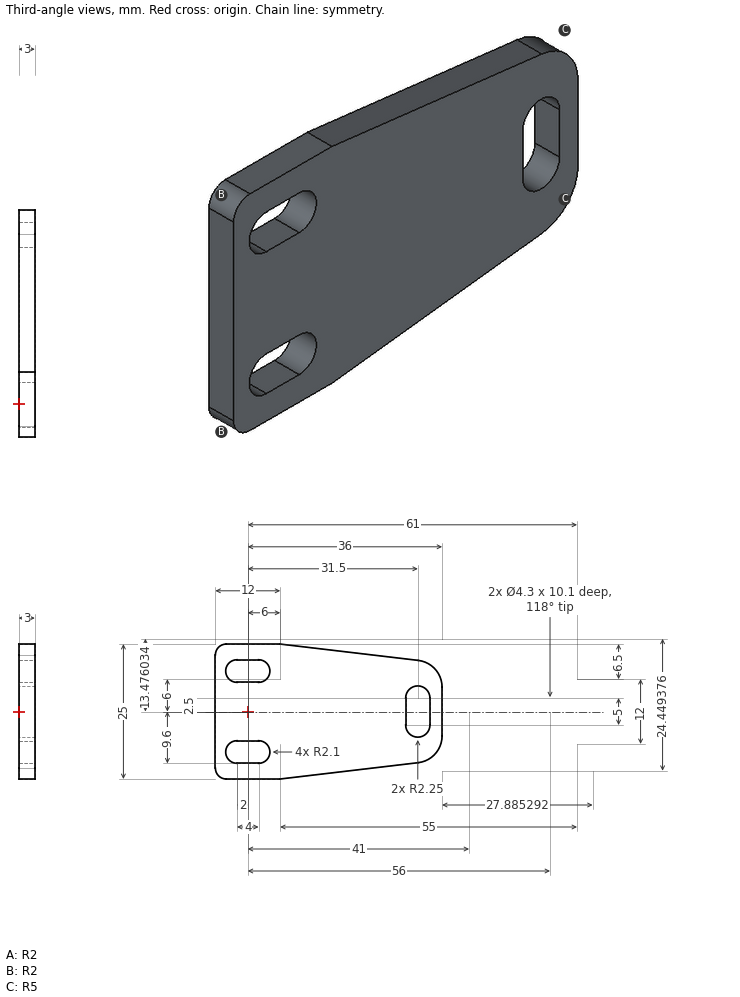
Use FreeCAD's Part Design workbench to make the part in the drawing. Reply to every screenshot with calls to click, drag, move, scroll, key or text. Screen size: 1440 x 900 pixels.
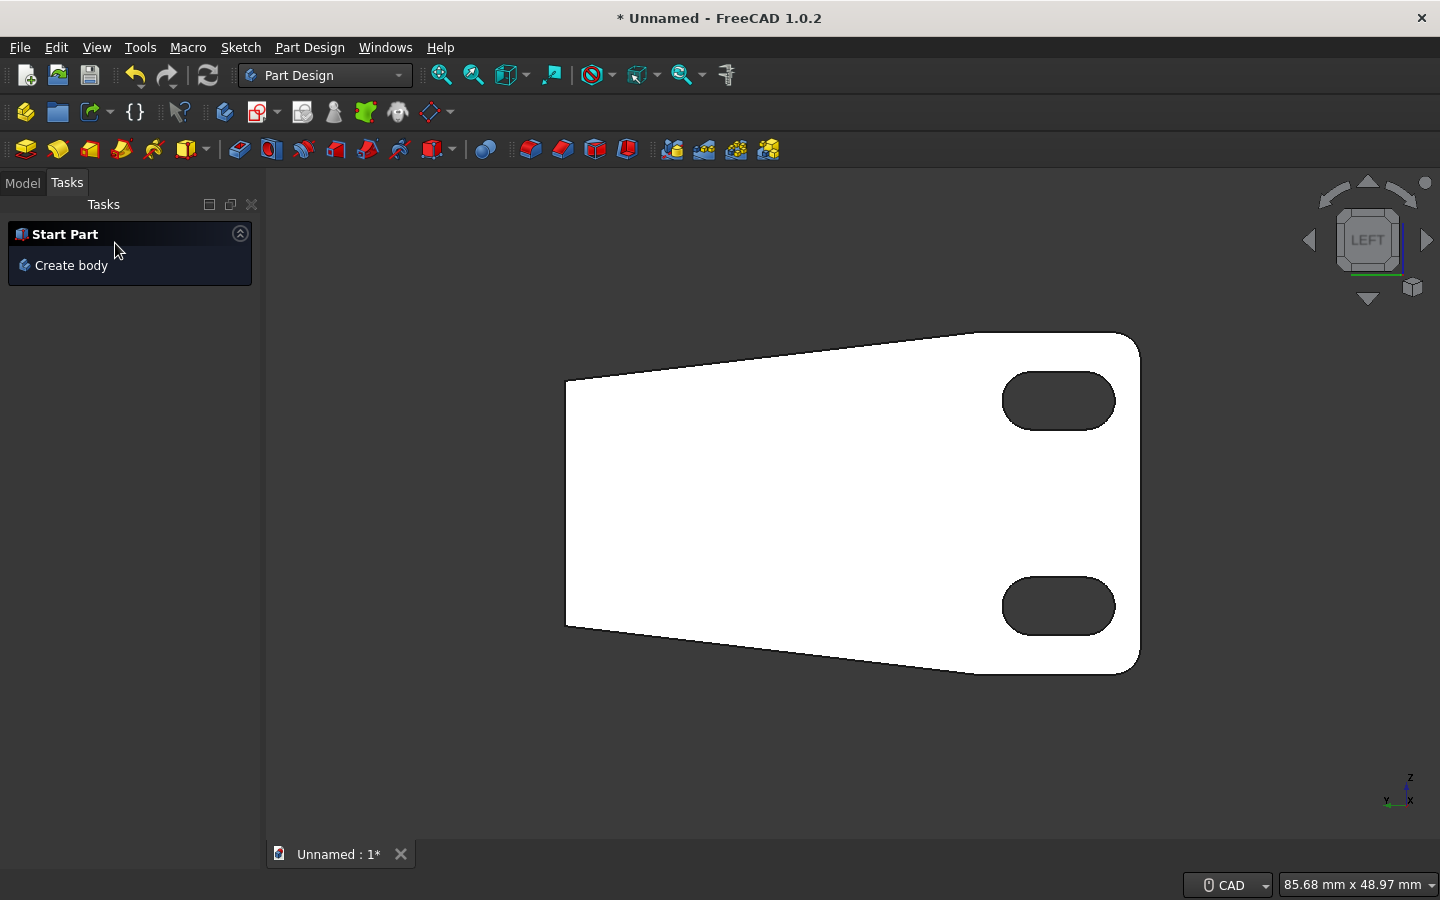
click(853, 502)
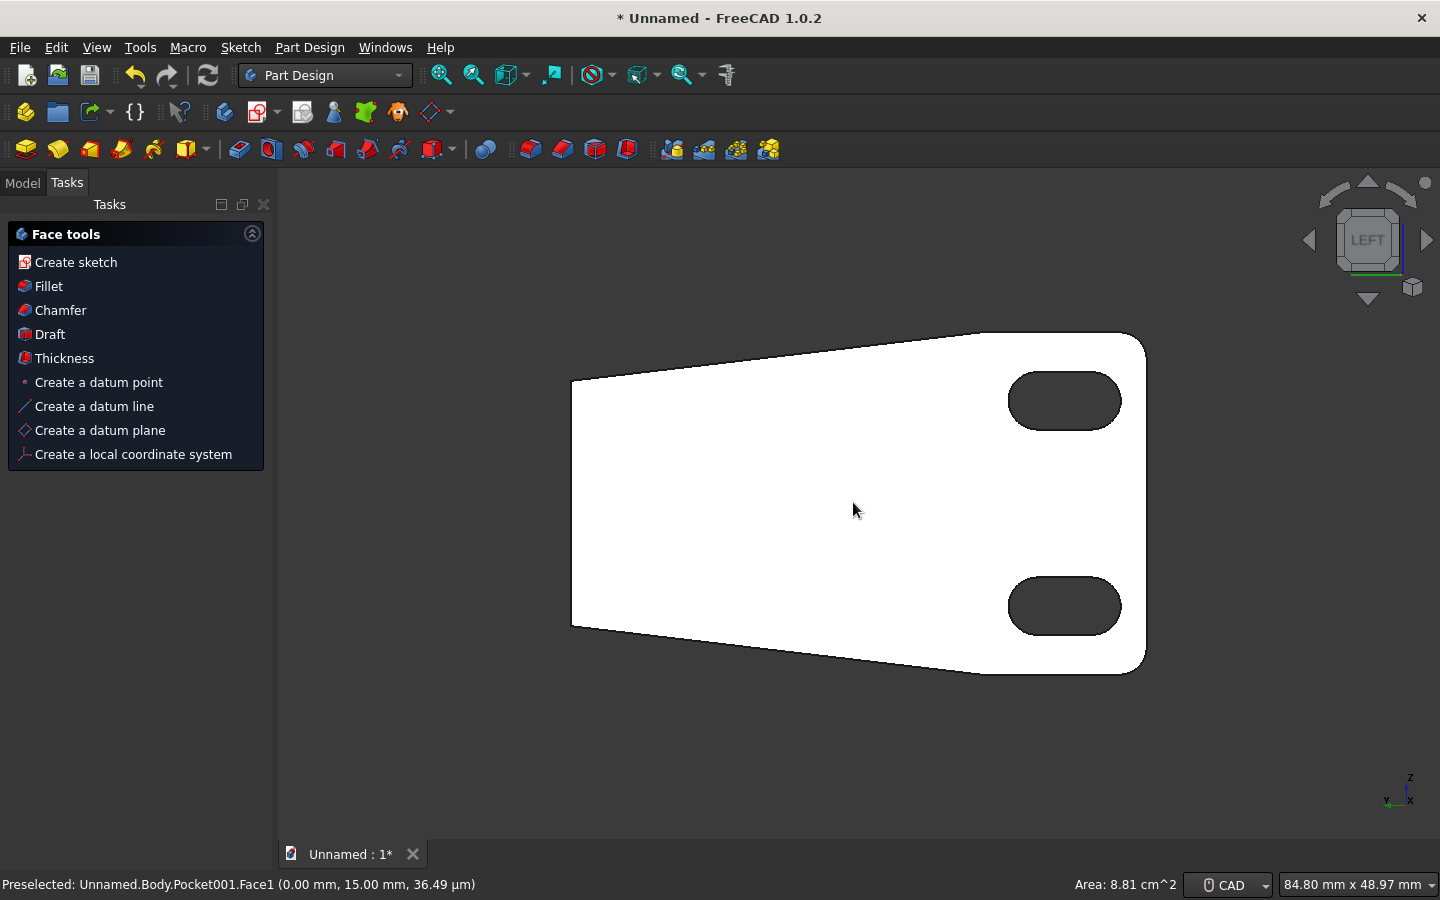
click(258, 112)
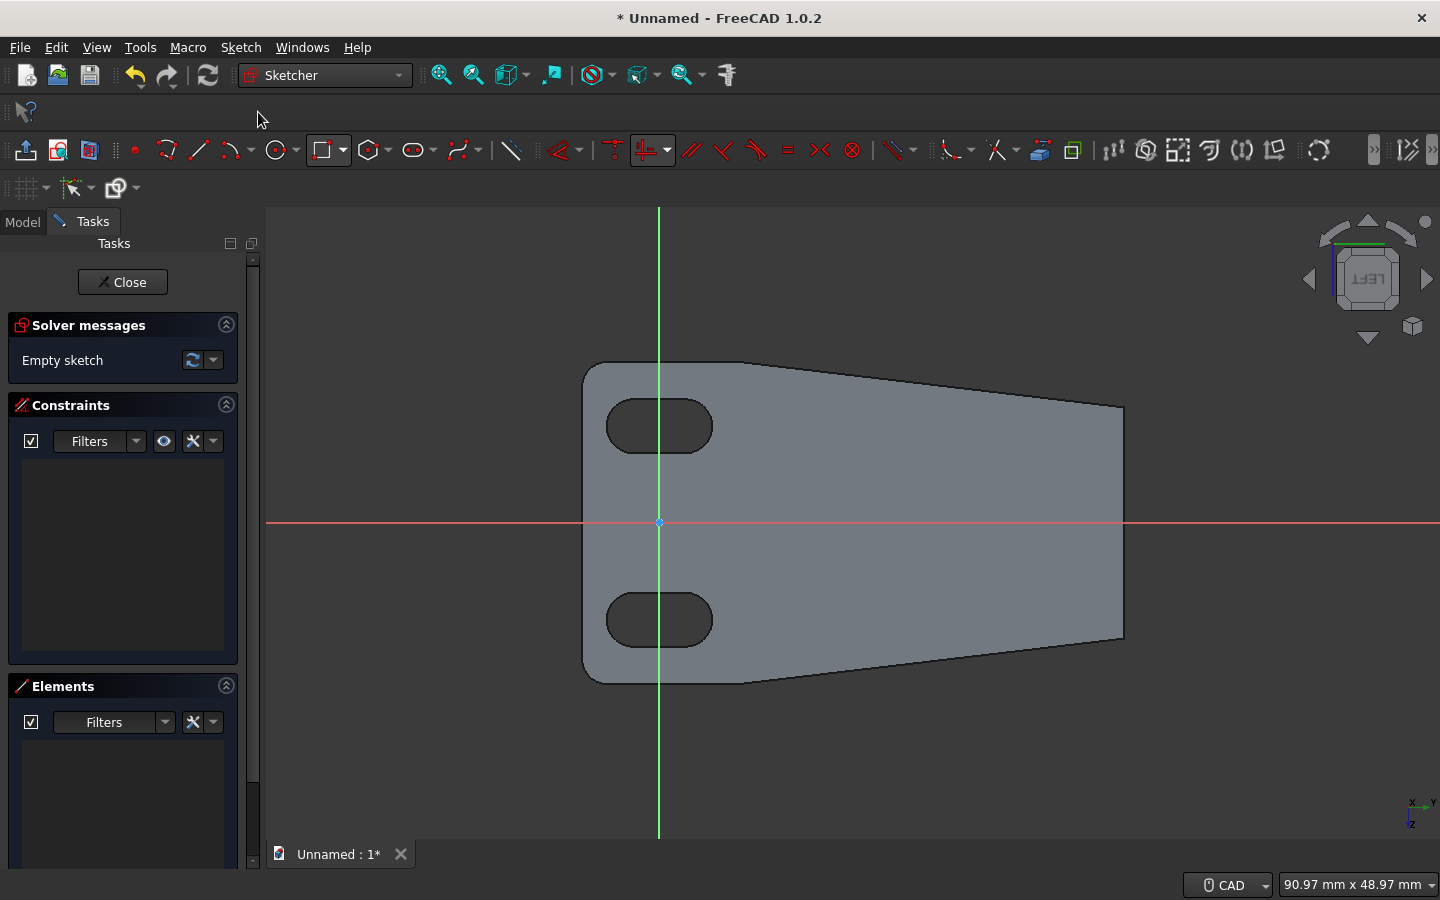
scroll(1187, 523, up, 6)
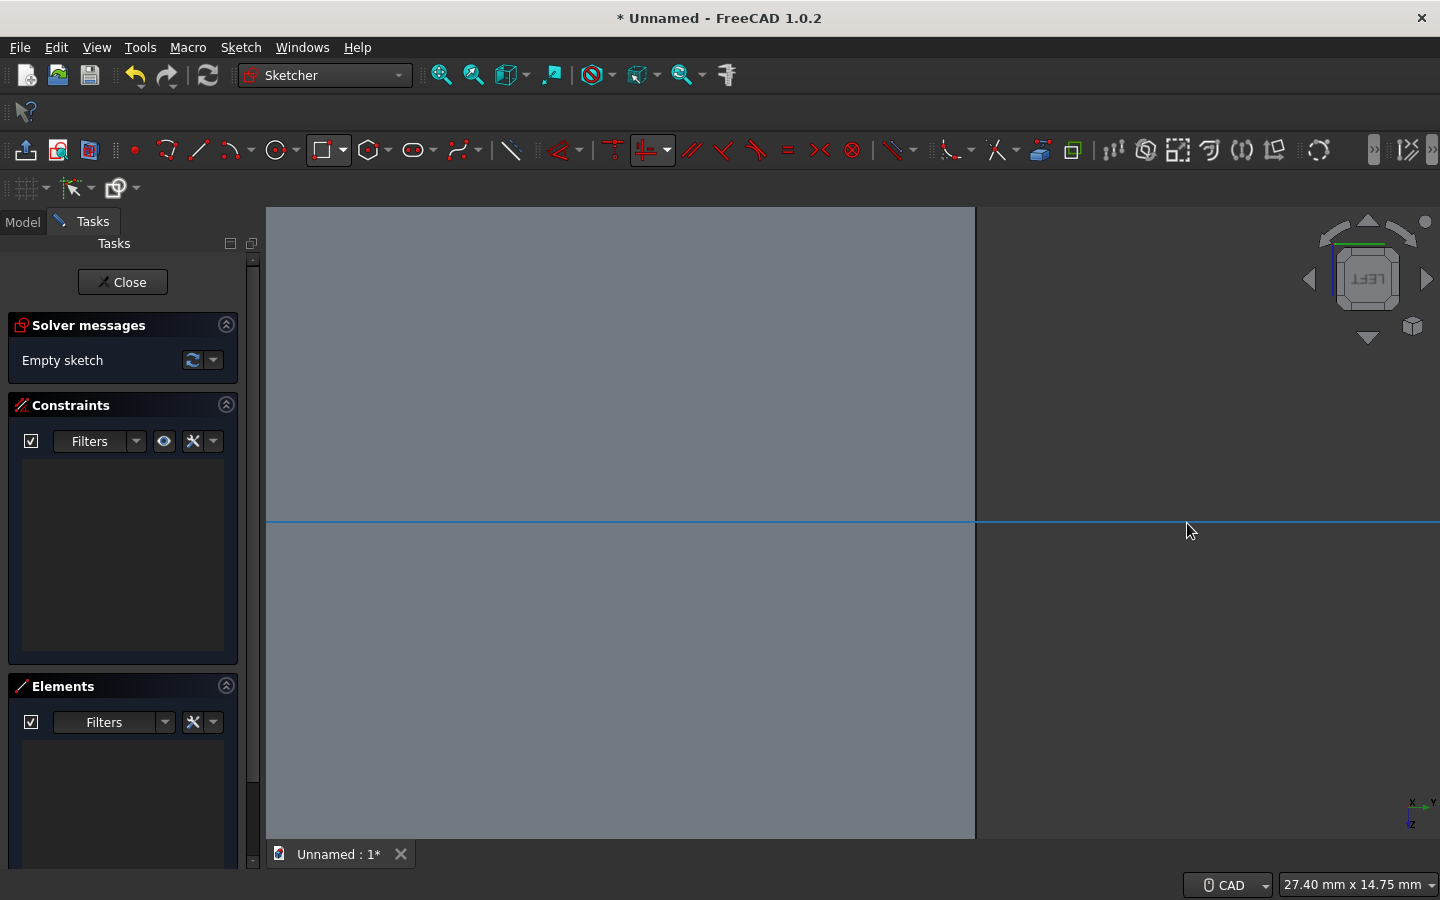
click(414, 150)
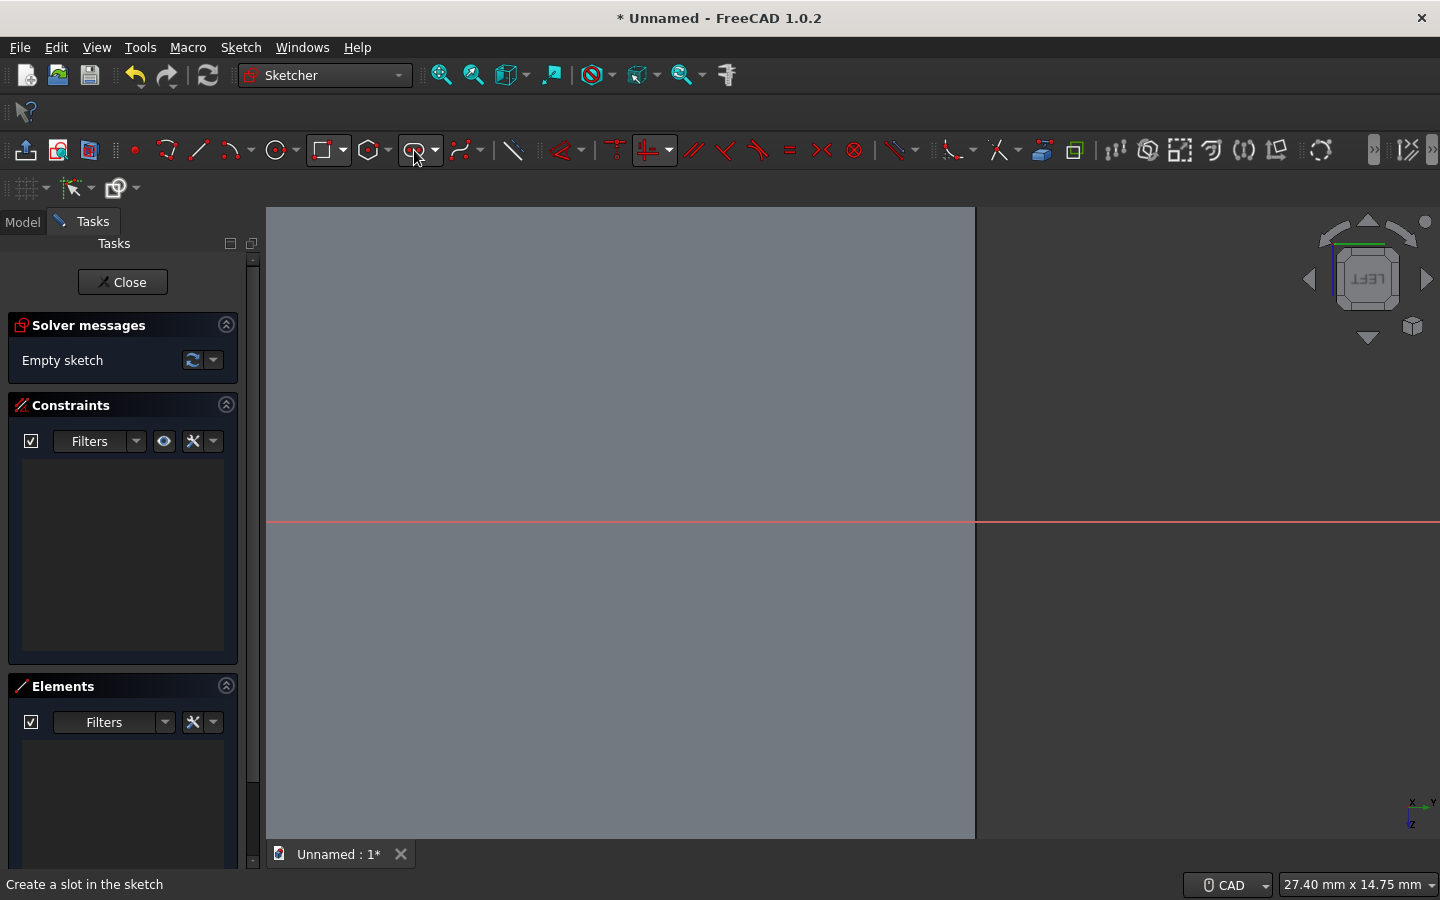
click(783, 629)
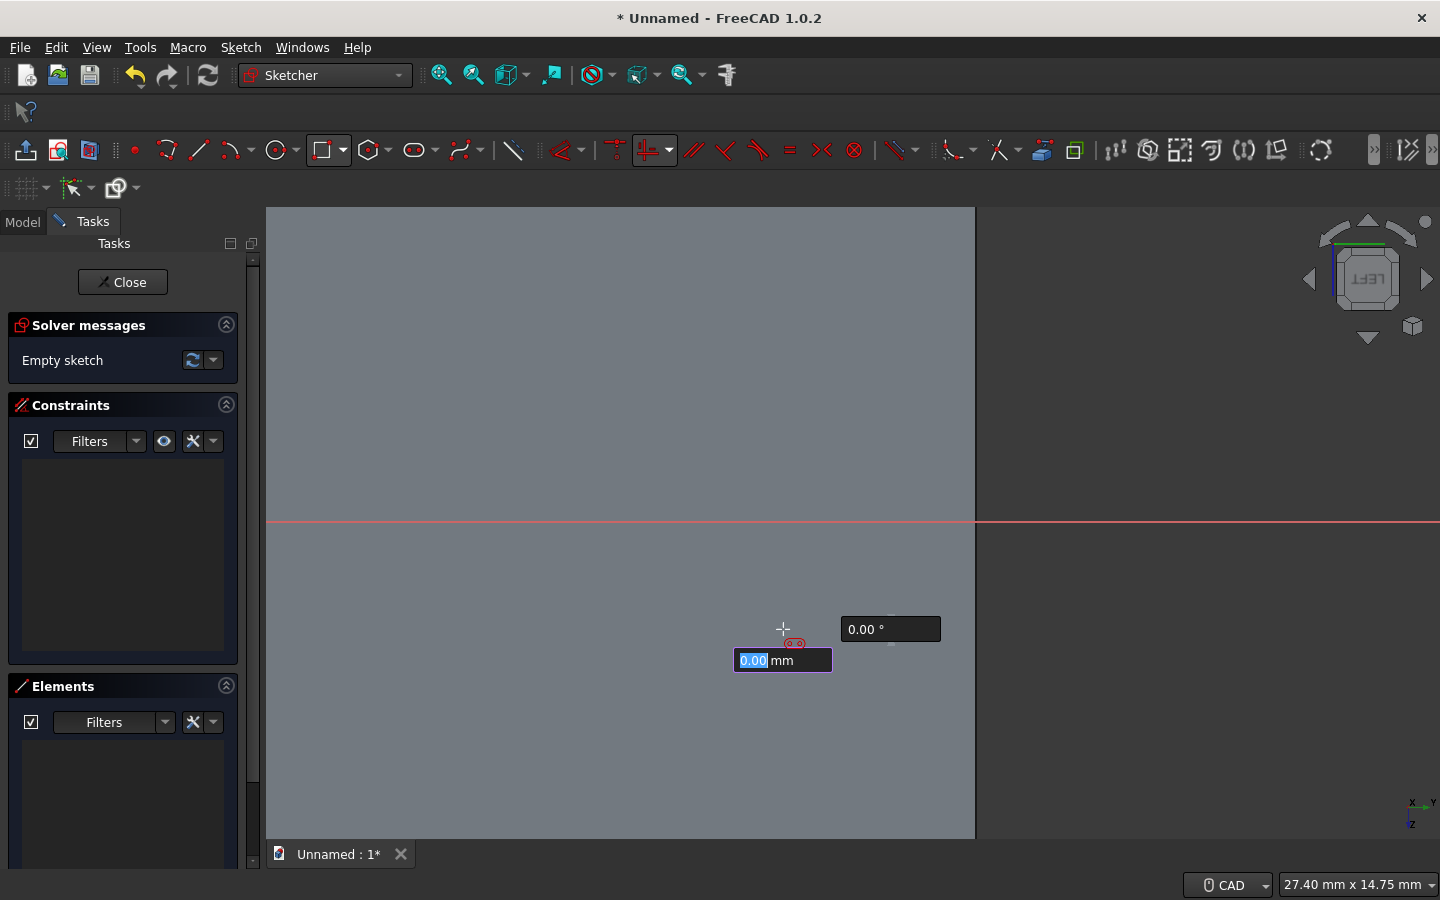
click(783, 415)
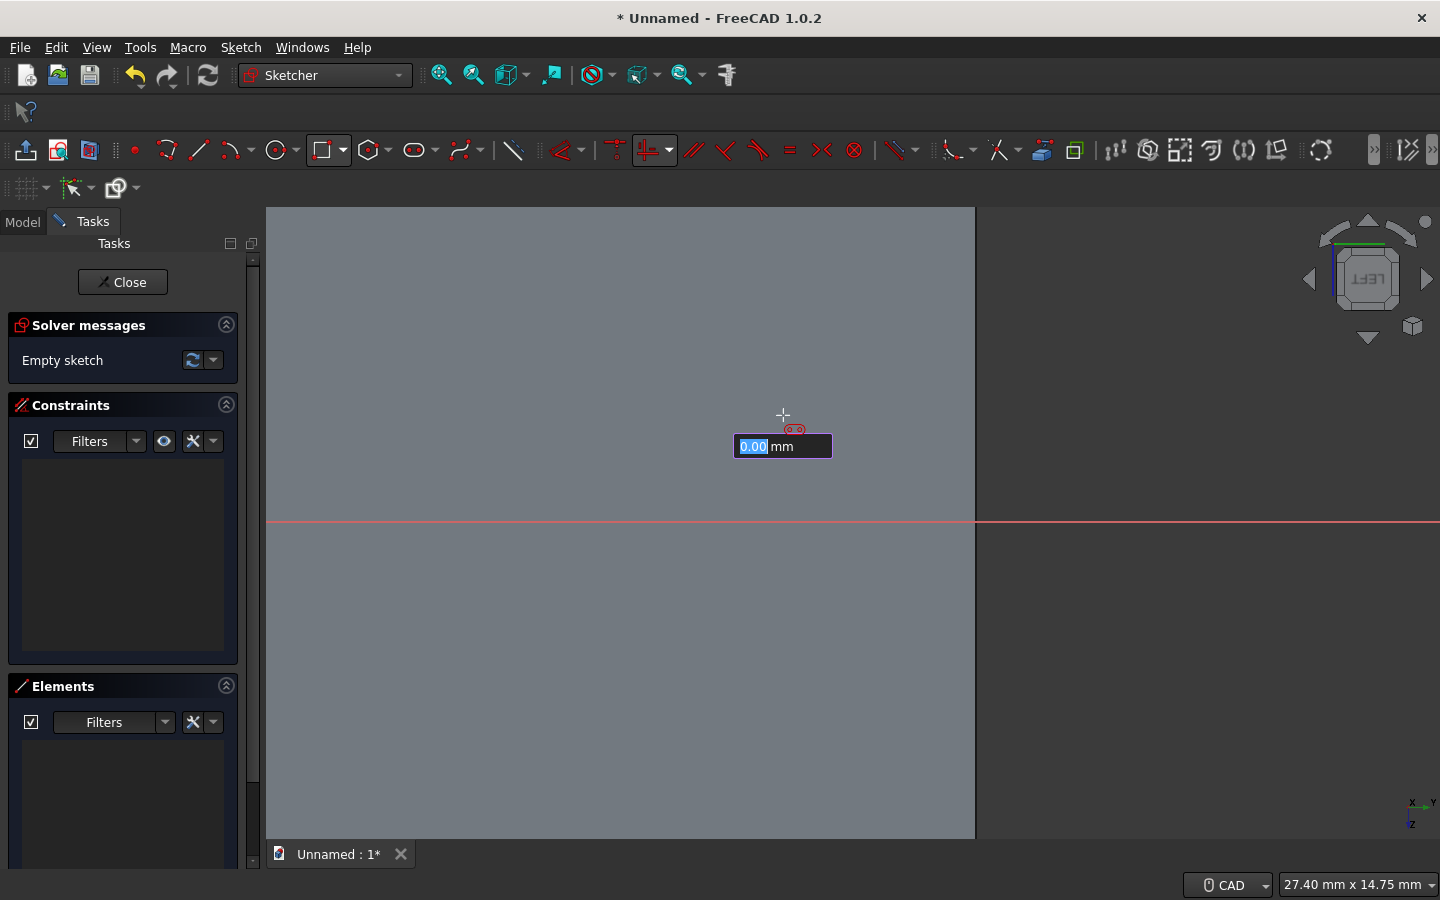
click(880, 554)
key(Escape)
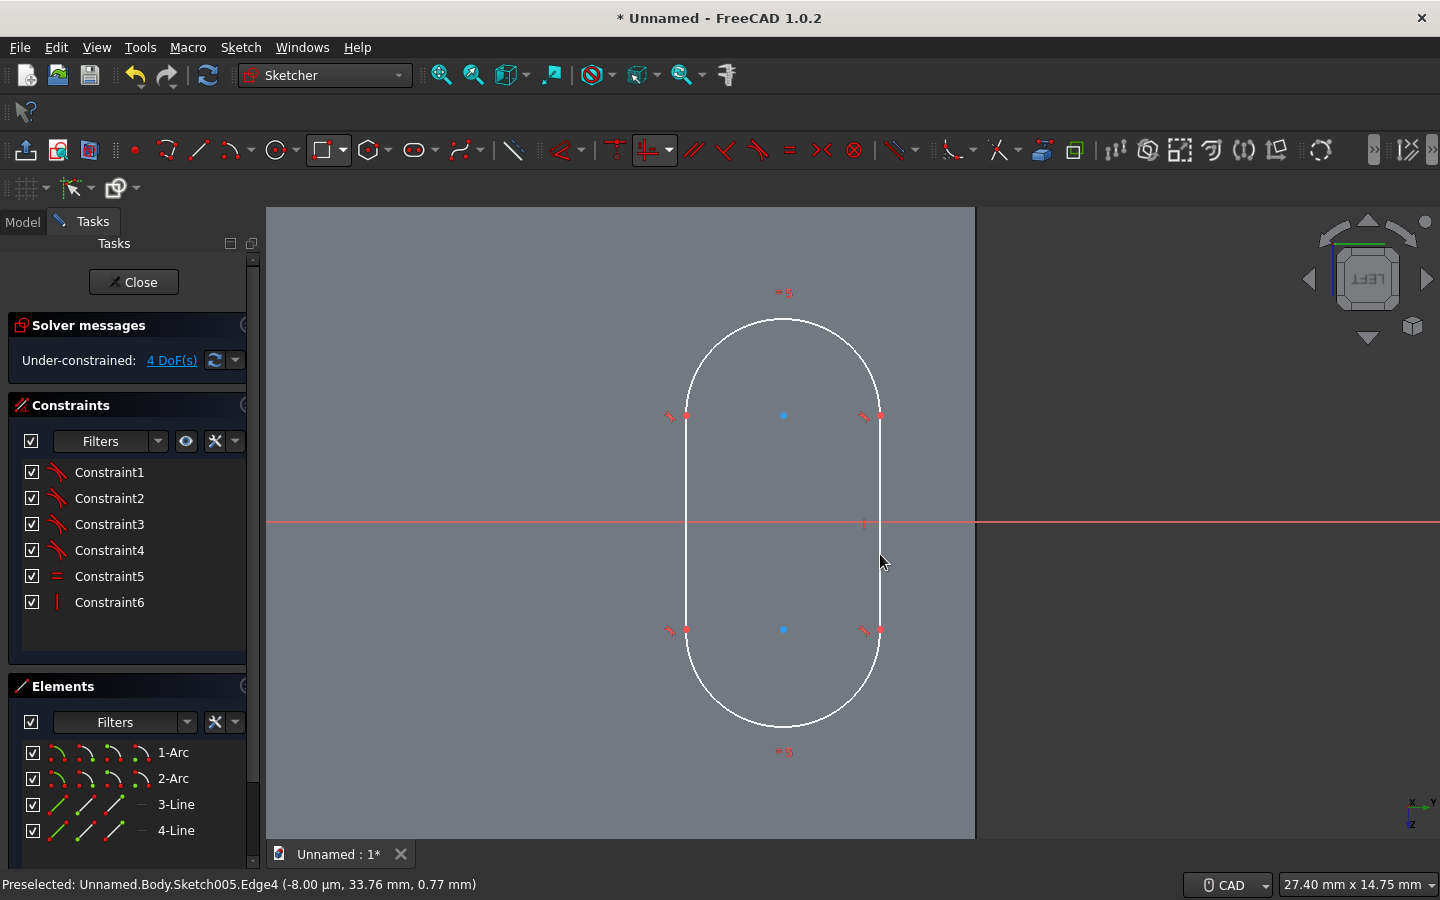
click(560, 150)